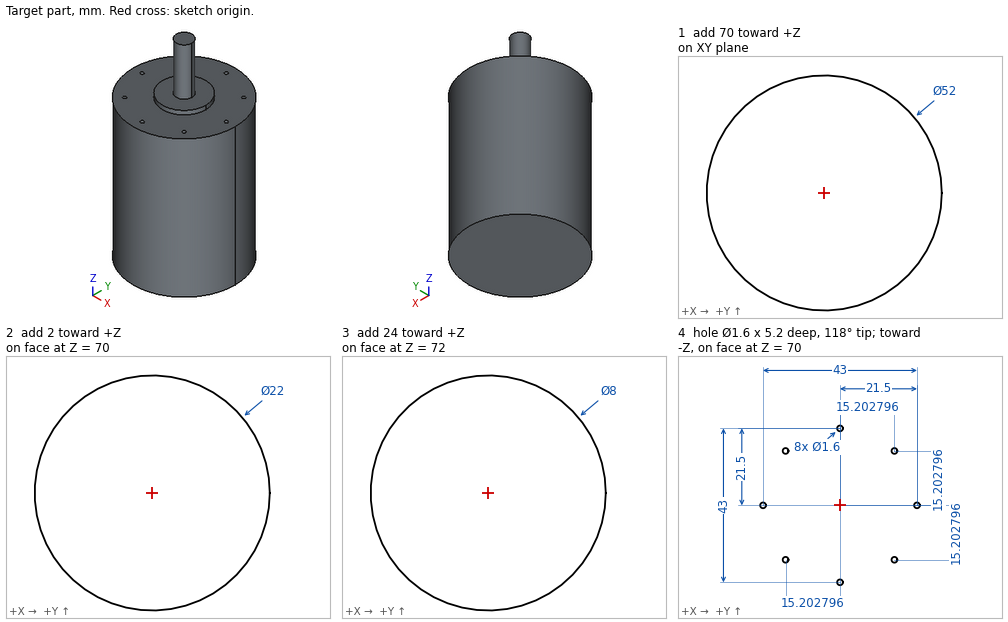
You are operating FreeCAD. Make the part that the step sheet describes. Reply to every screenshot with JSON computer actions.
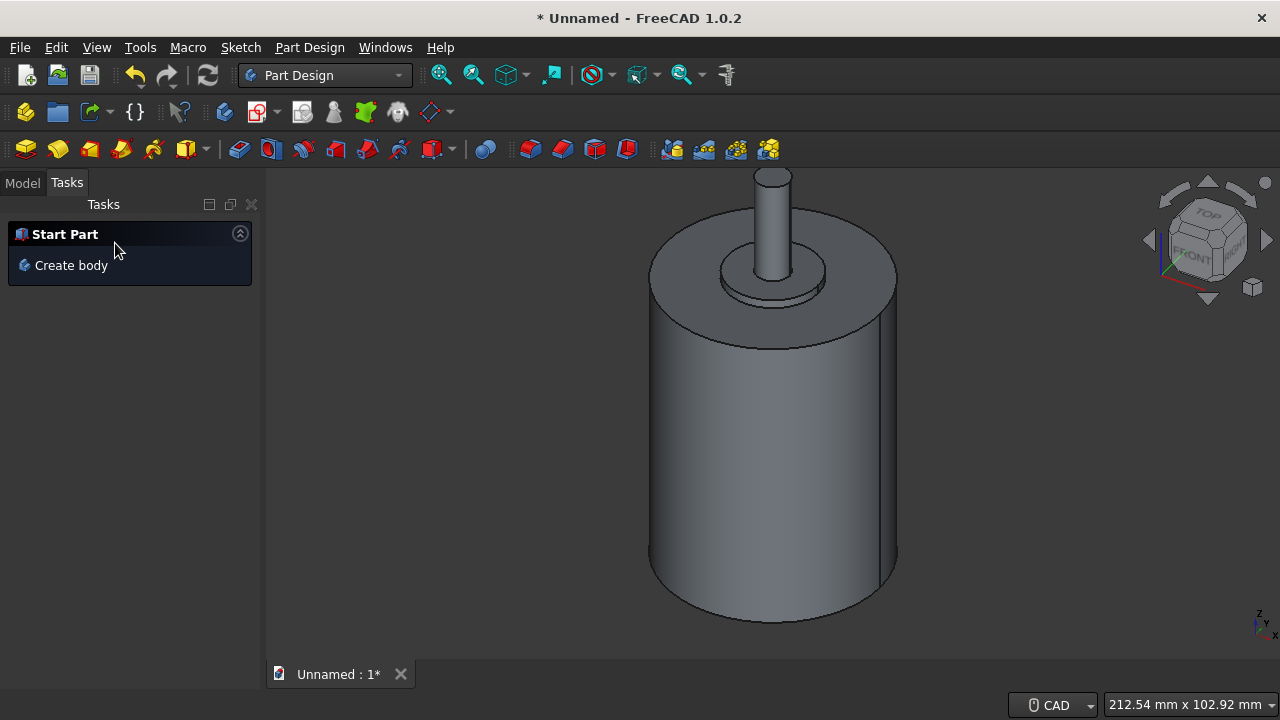
{"action": "key", "text": "v f"}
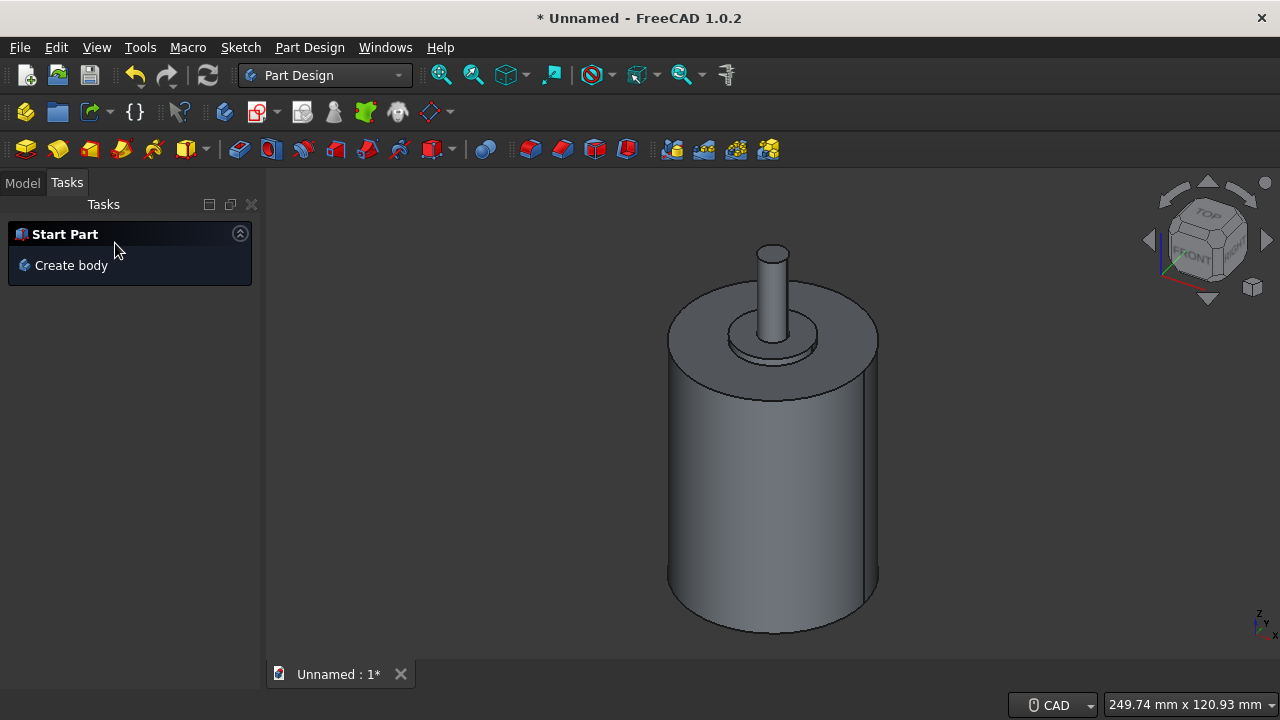
{"action": "left_click", "coordinate": [717, 361]}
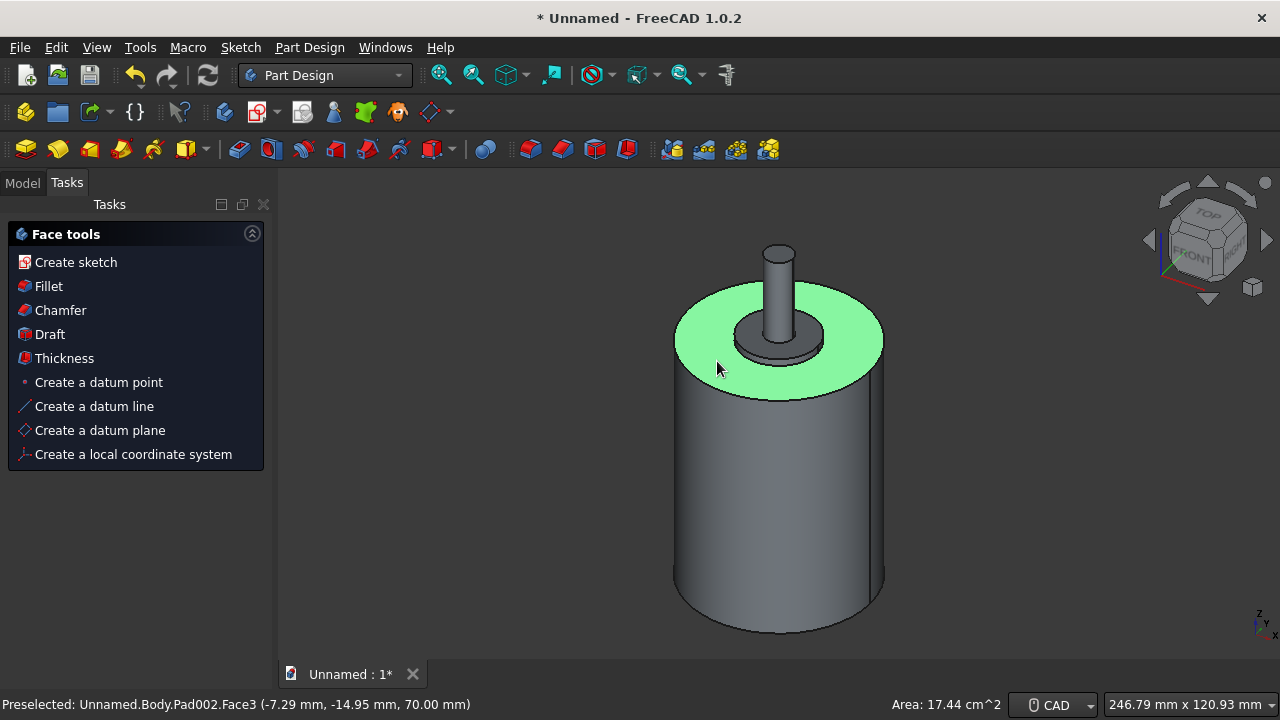
{"action": "left_click", "coordinate": [258, 112]}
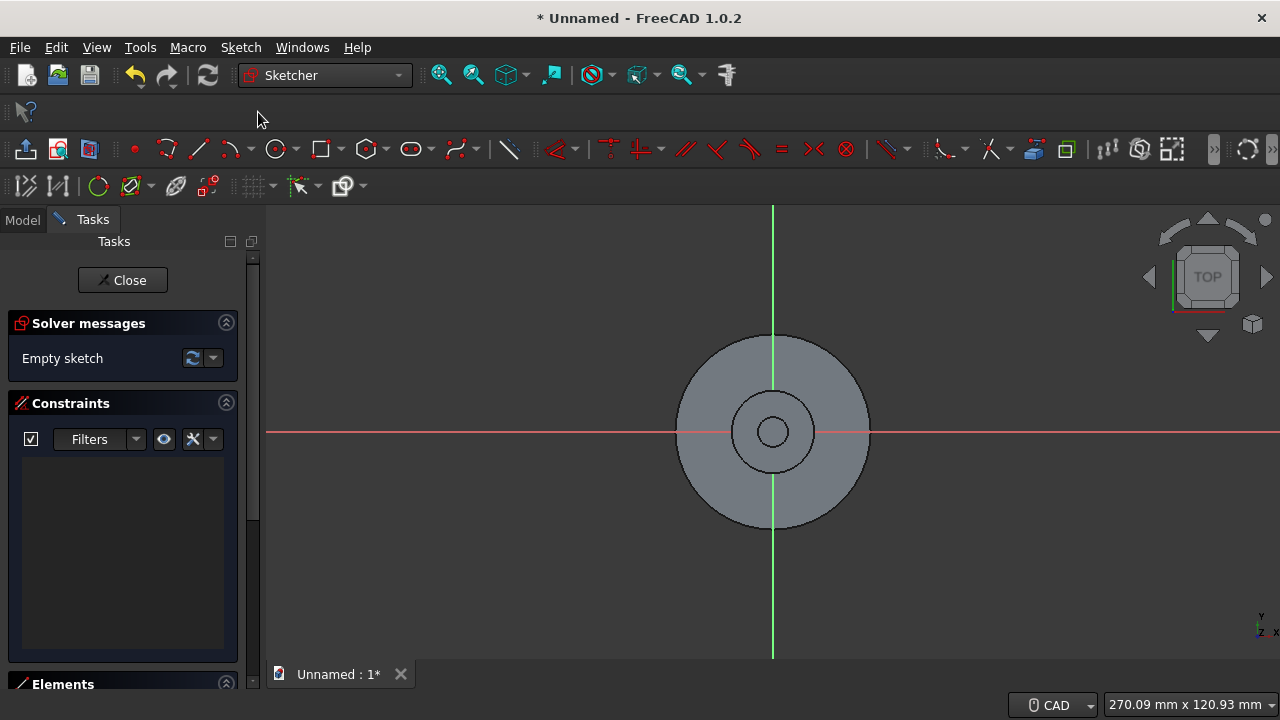
{"action": "scroll", "coordinate": [856, 432], "scroll_direction": "up", "scroll_amount": 3}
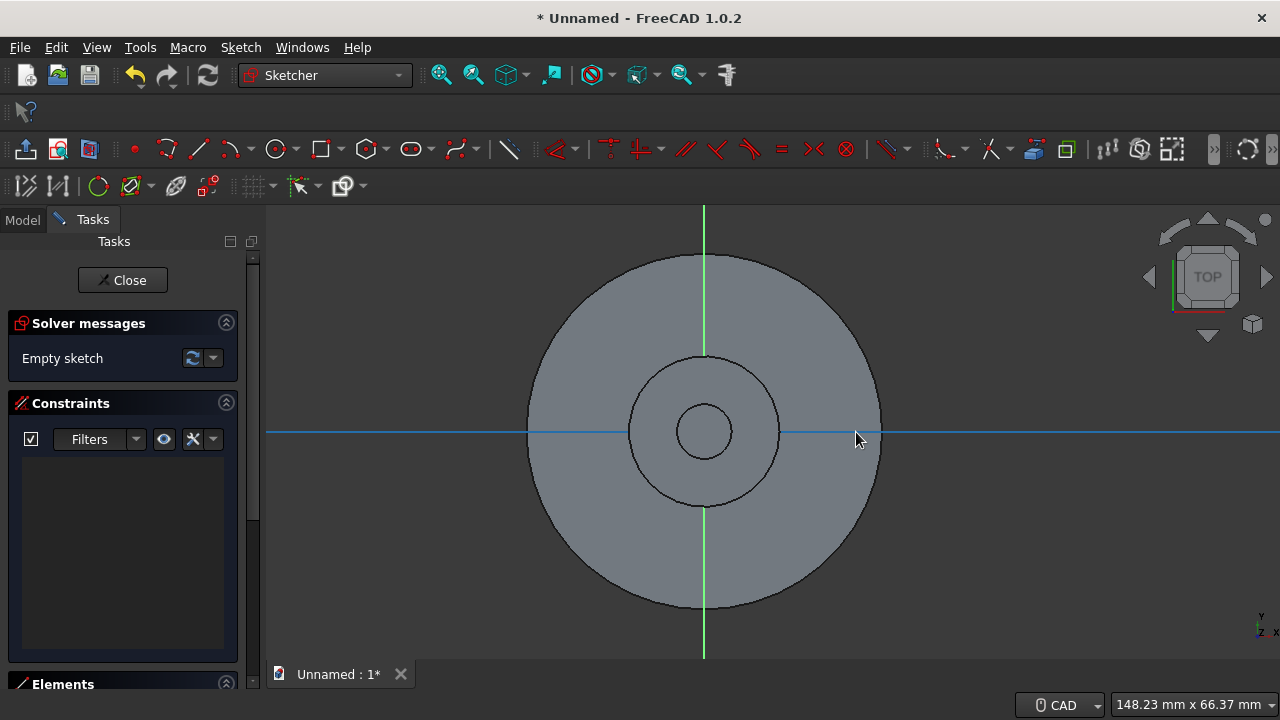
{"action": "left_click", "coordinate": [276, 150]}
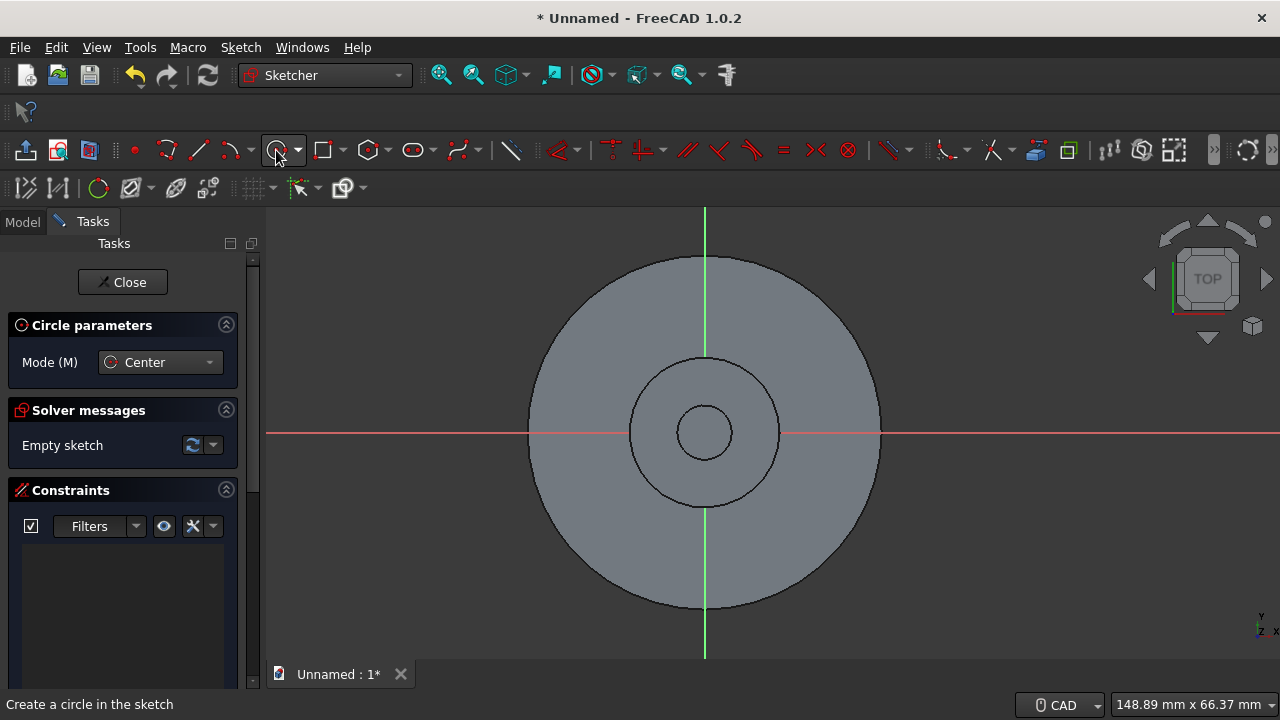
{"action": "scroll", "coordinate": [705, 286], "scroll_direction": "up", "scroll_amount": 8}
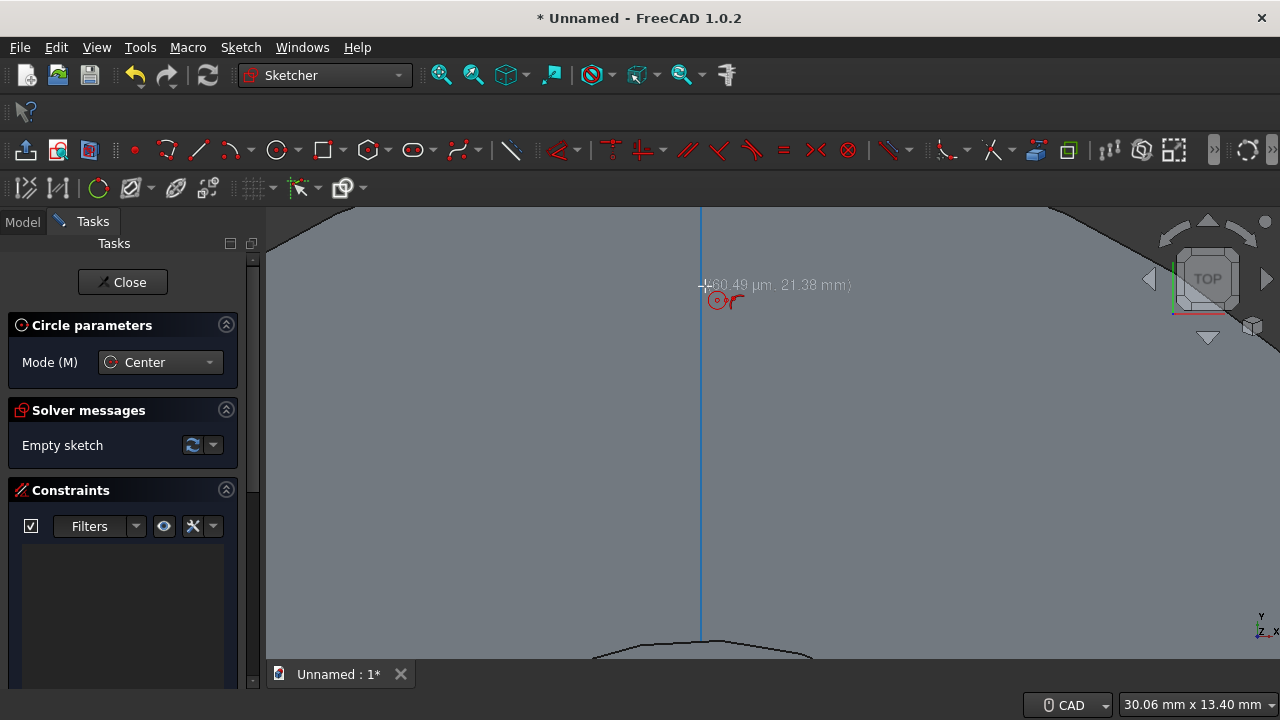
{"action": "scroll", "coordinate": [705, 287], "scroll_direction": "down", "scroll_amount": 8}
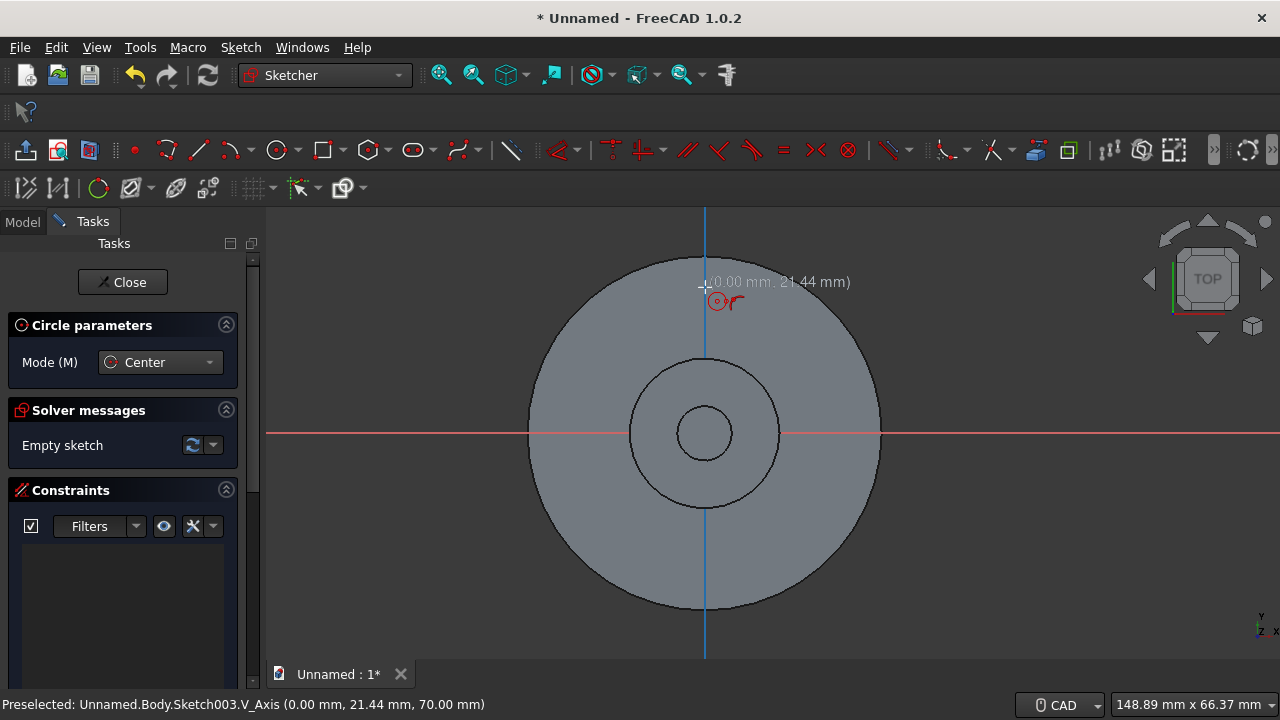
{"action": "left_click", "coordinate": [705, 287]}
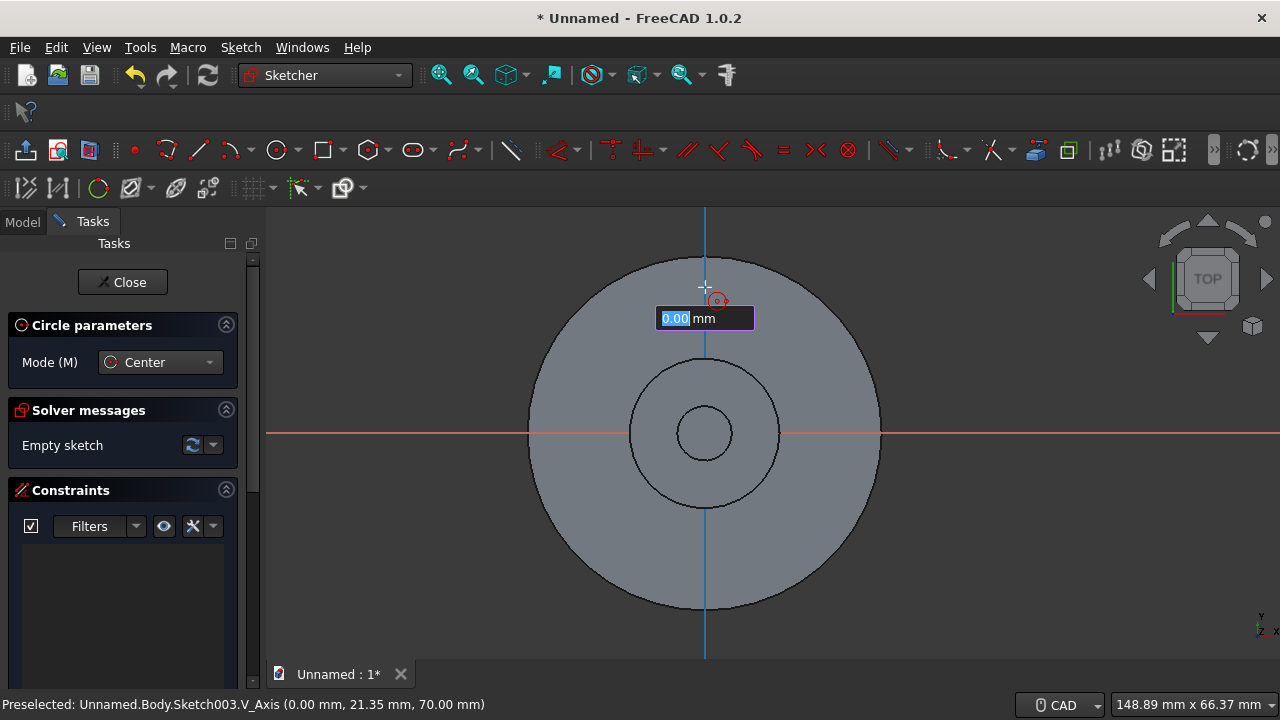
{"action": "scroll", "coordinate": [710, 285], "scroll_direction": "up", "scroll_amount": 6}
{"action": "mouse_move", "coordinate": [708, 285]}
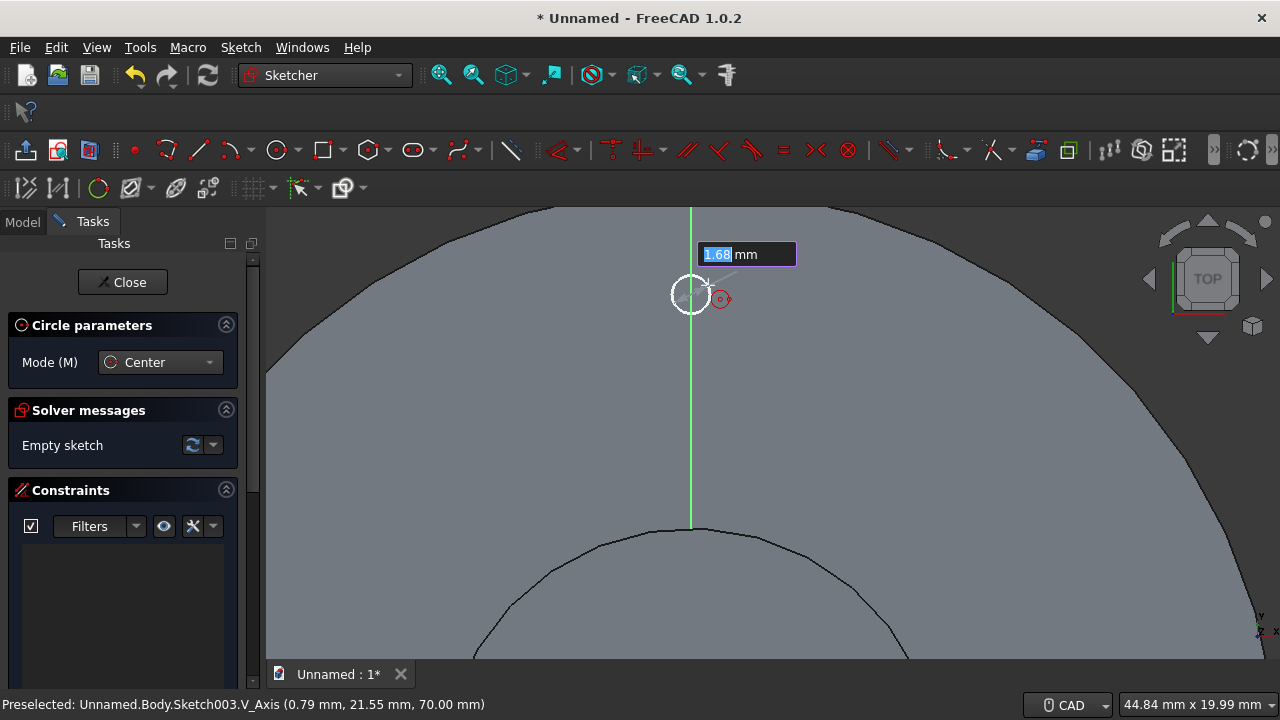
{"action": "type", "text": "1.6"}
{"action": "key", "text": "Return"}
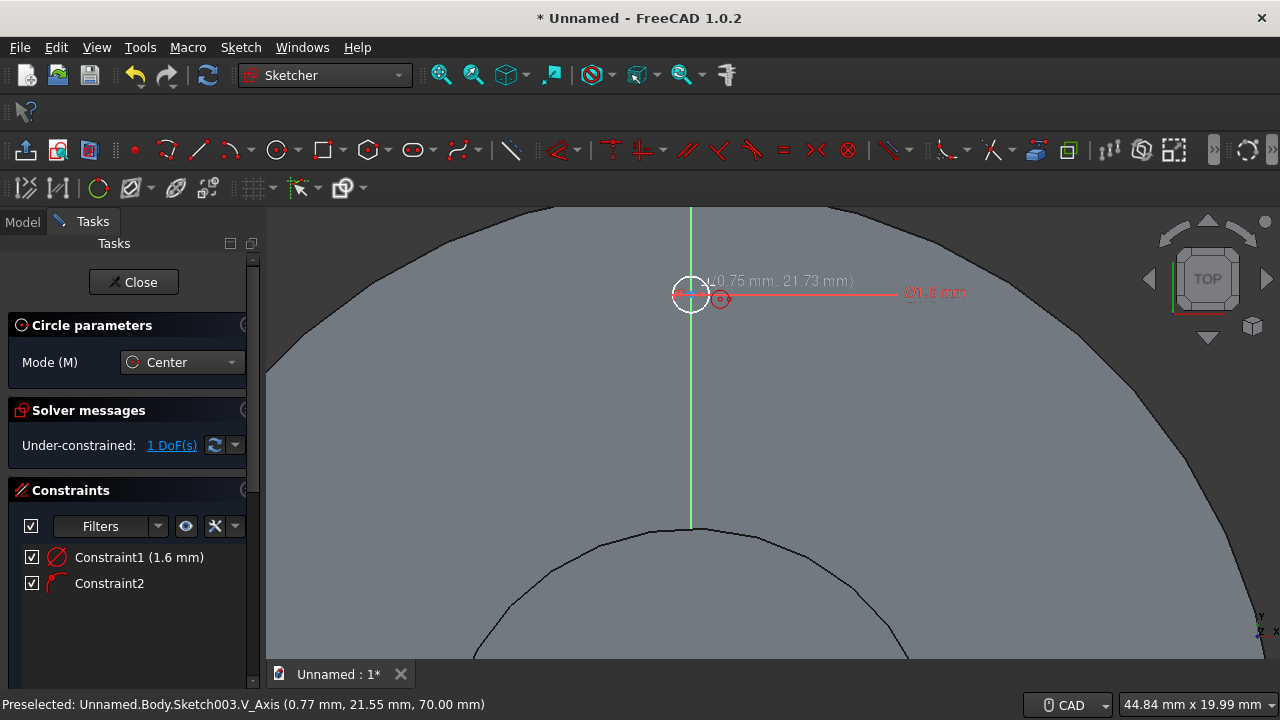
{"action": "scroll", "coordinate": [1035, 434], "scroll_direction": "up", "scroll_amount": 2}